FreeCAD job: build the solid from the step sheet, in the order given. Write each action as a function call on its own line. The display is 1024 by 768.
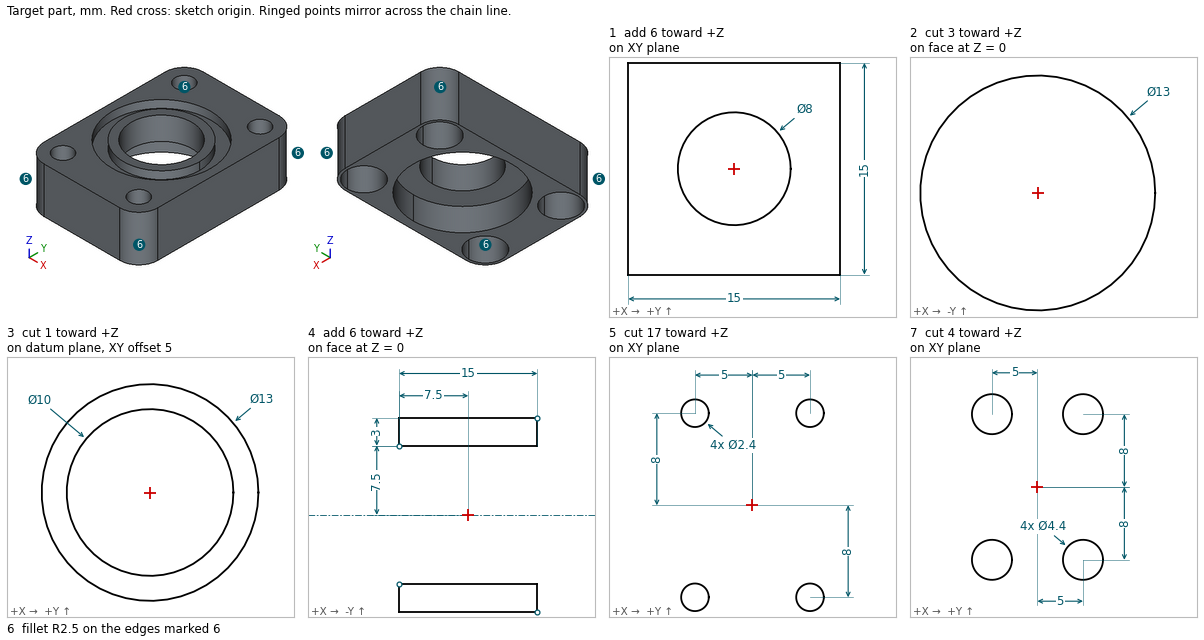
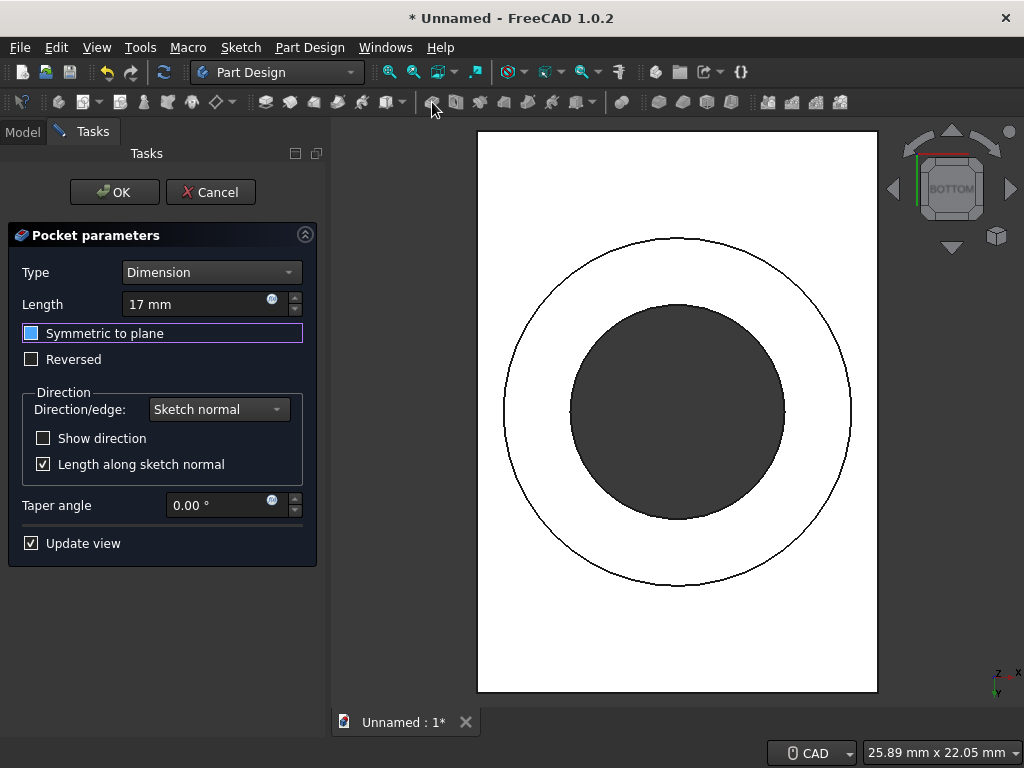
click(30, 359)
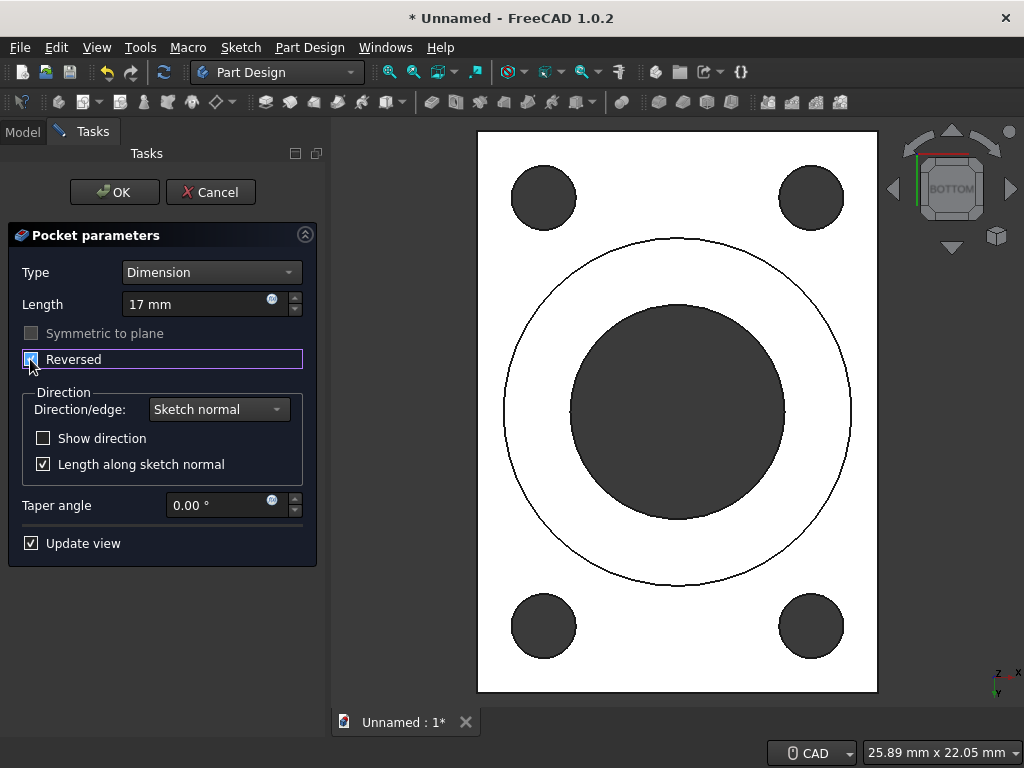
click(115, 192)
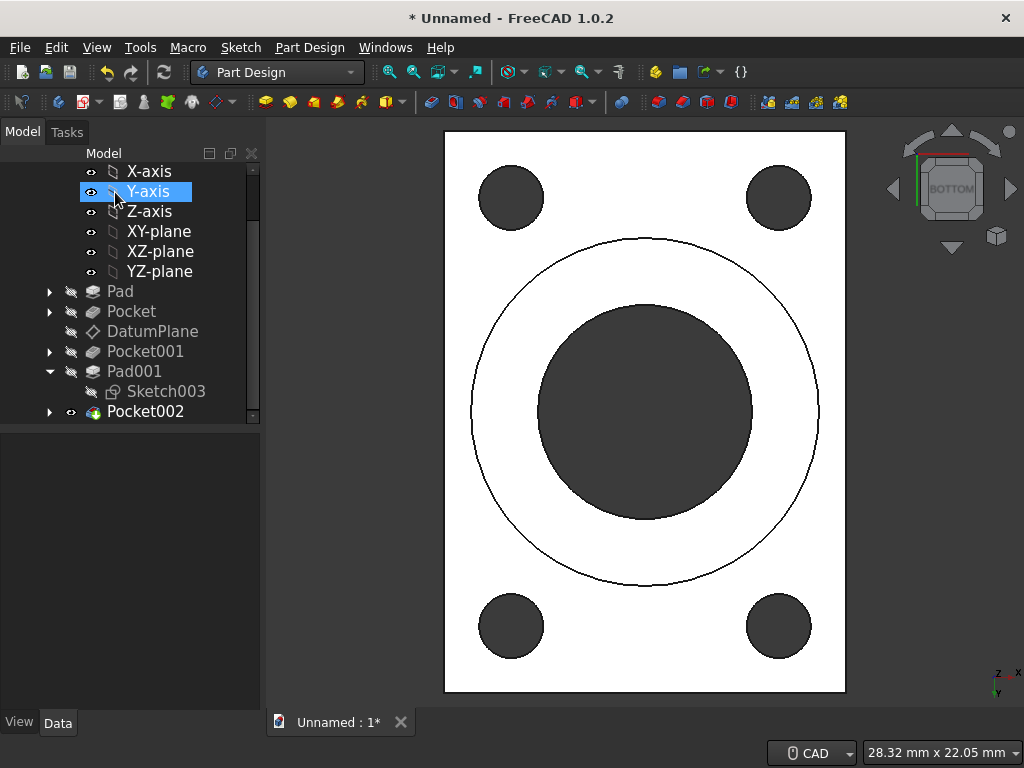
key(0)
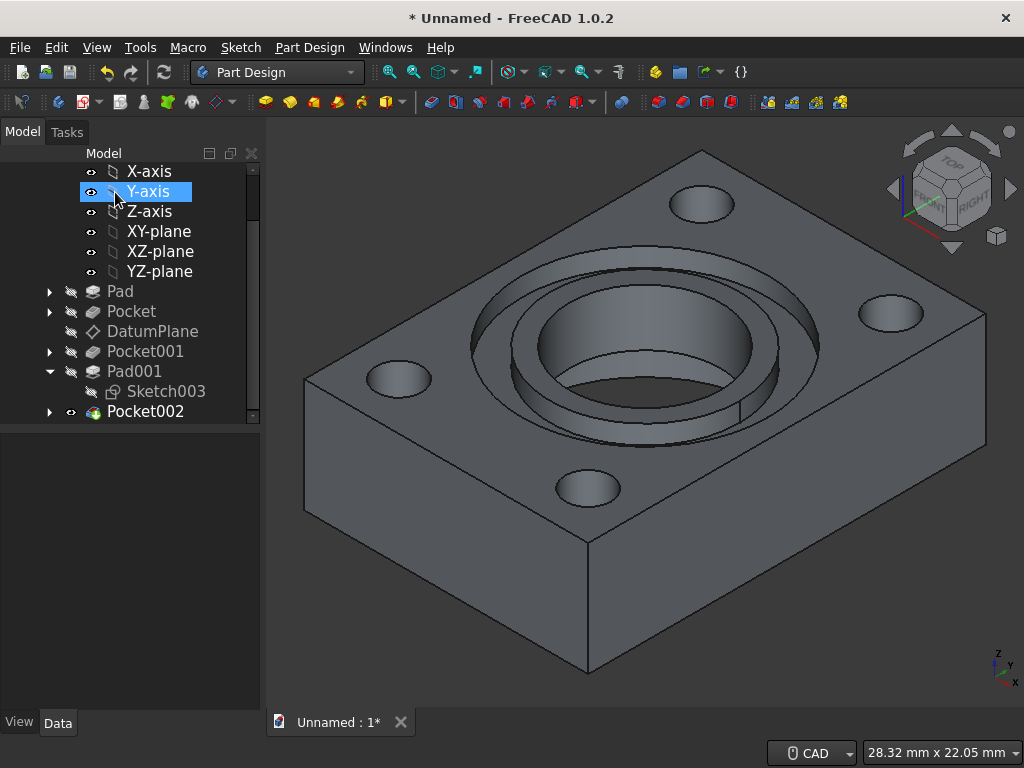
click(588, 608)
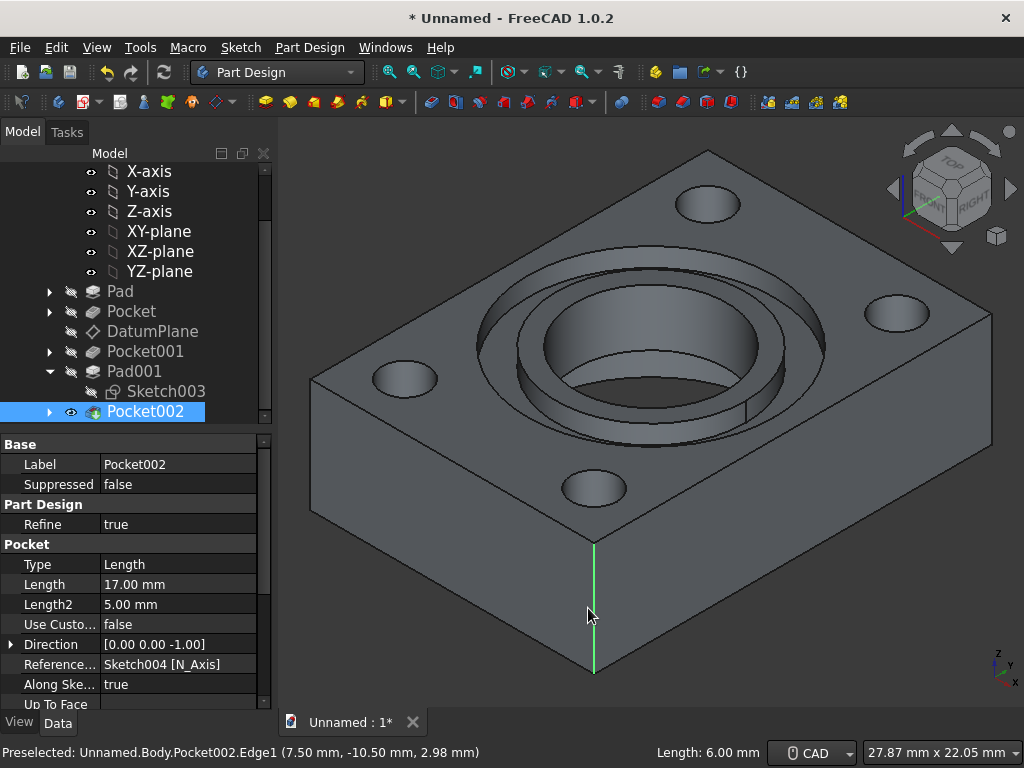
key(2)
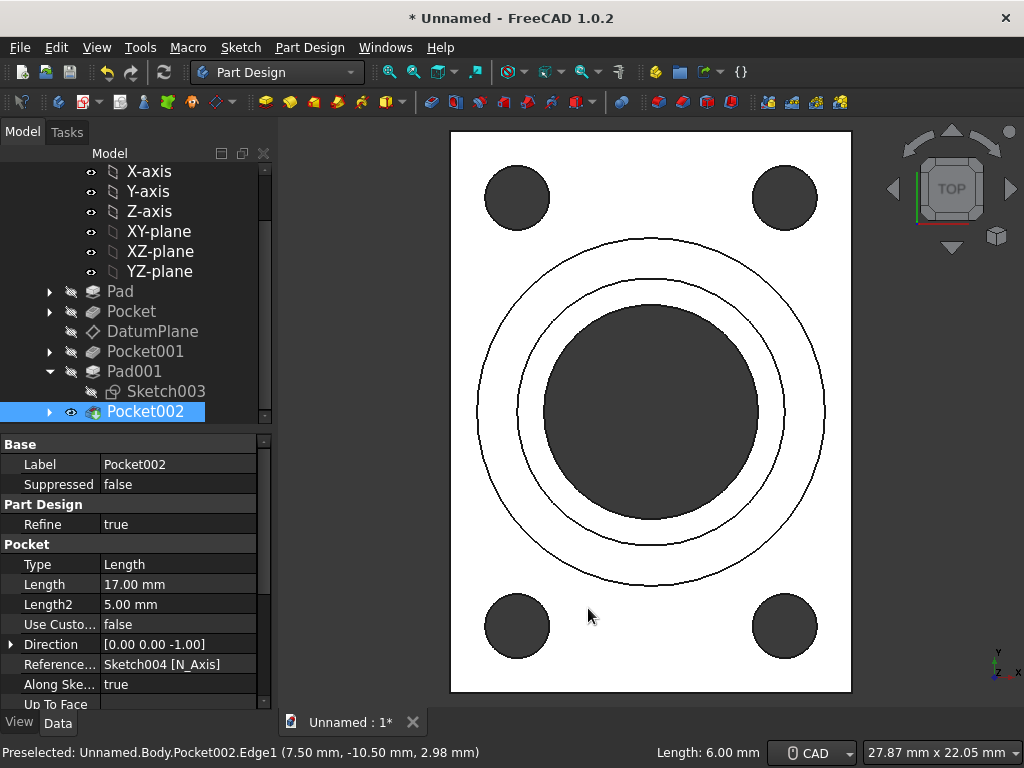
key(1)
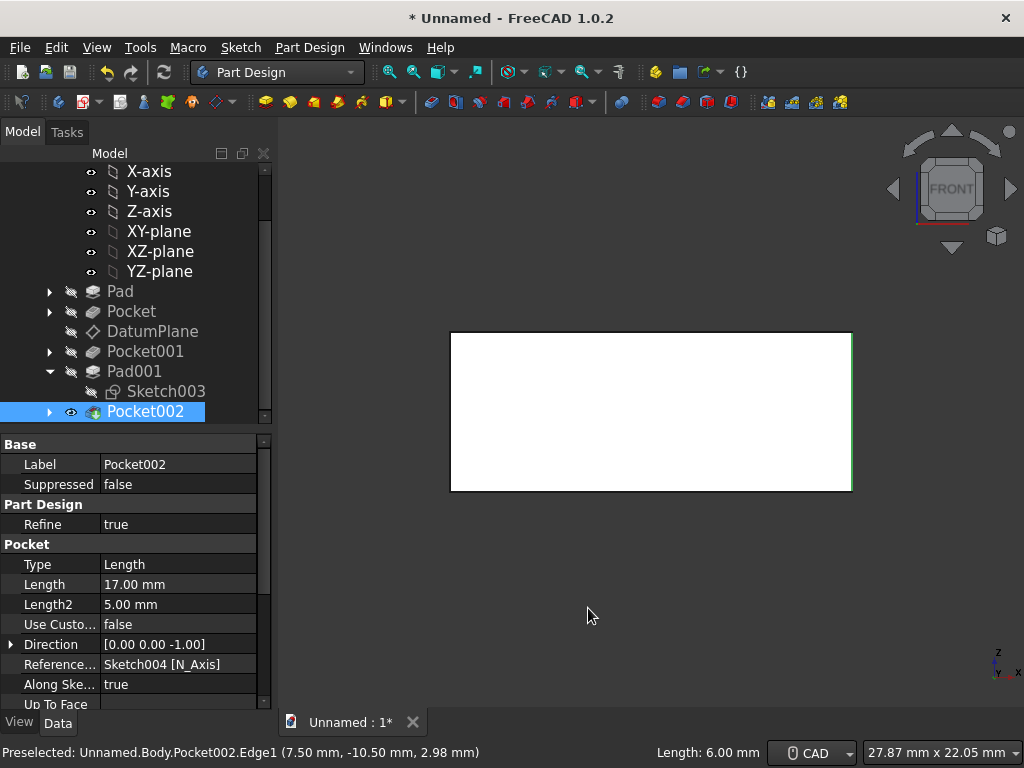
click(450, 411, ctrl)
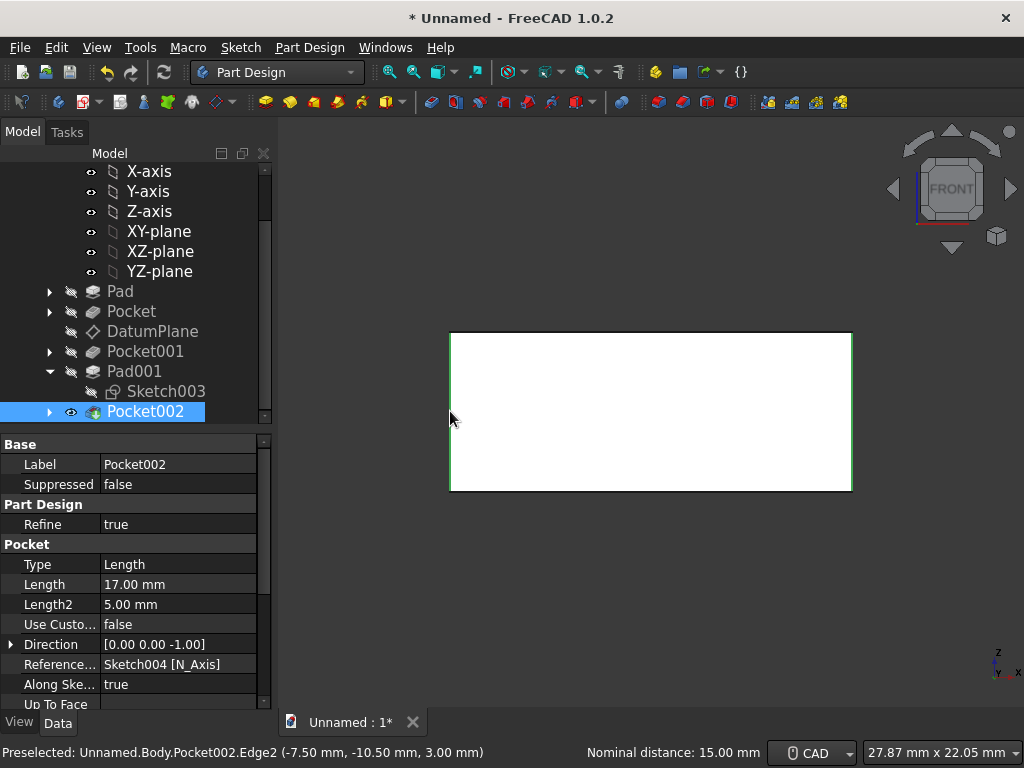
key(3)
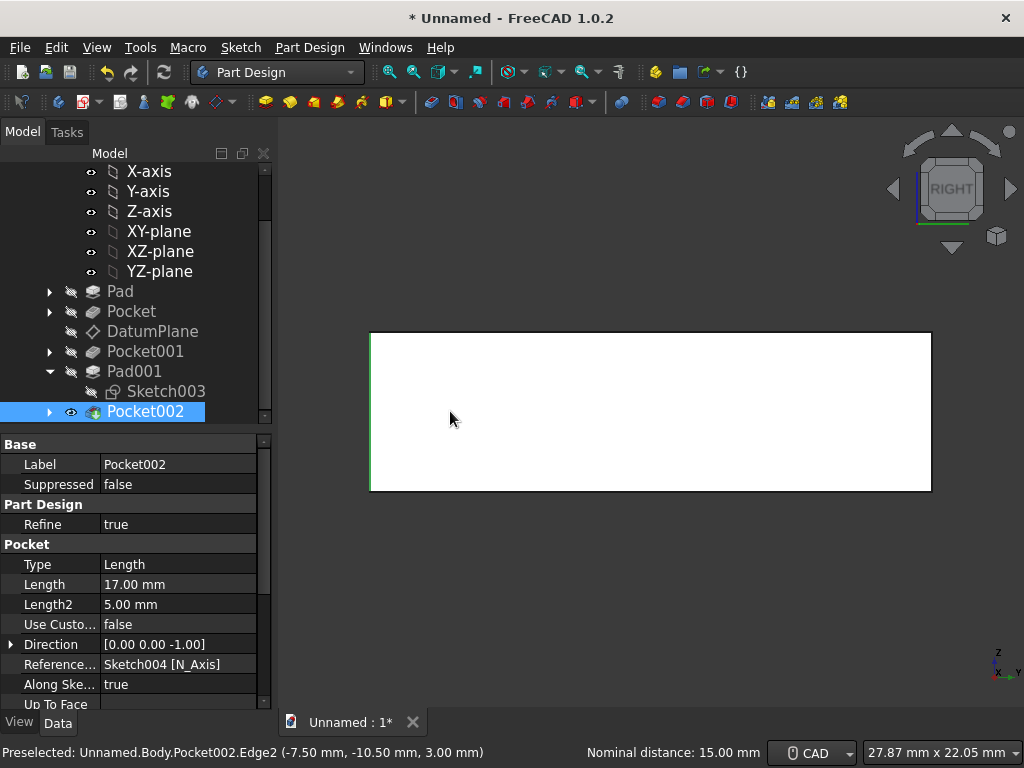
click(932, 411, ctrl)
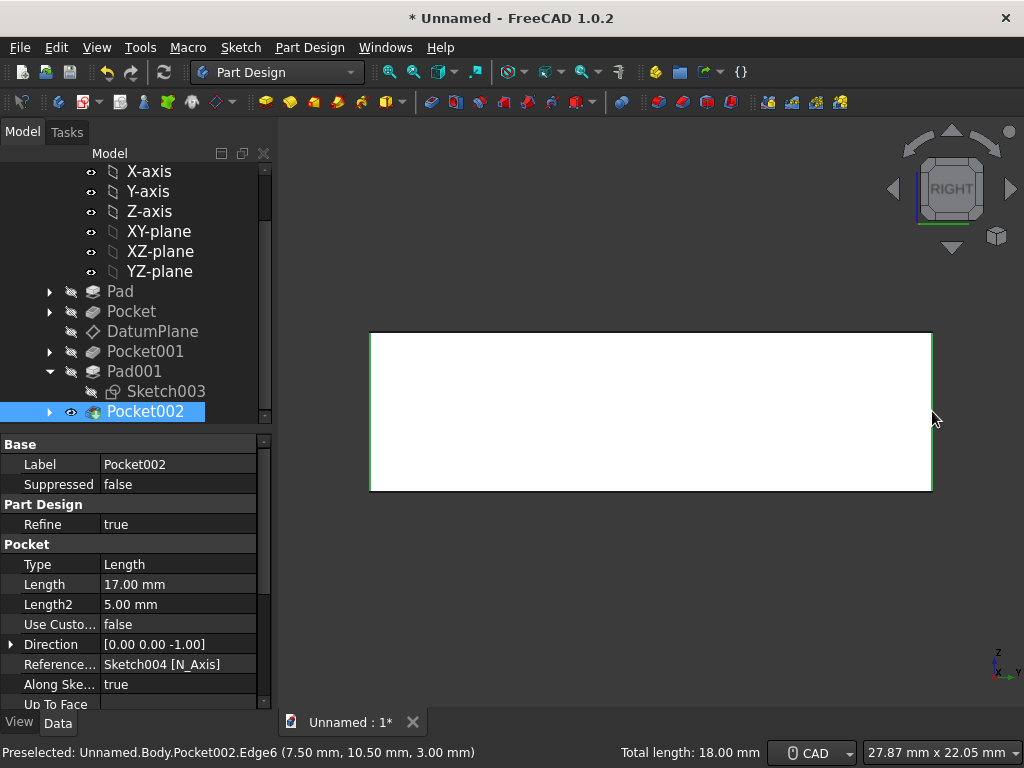
key(5)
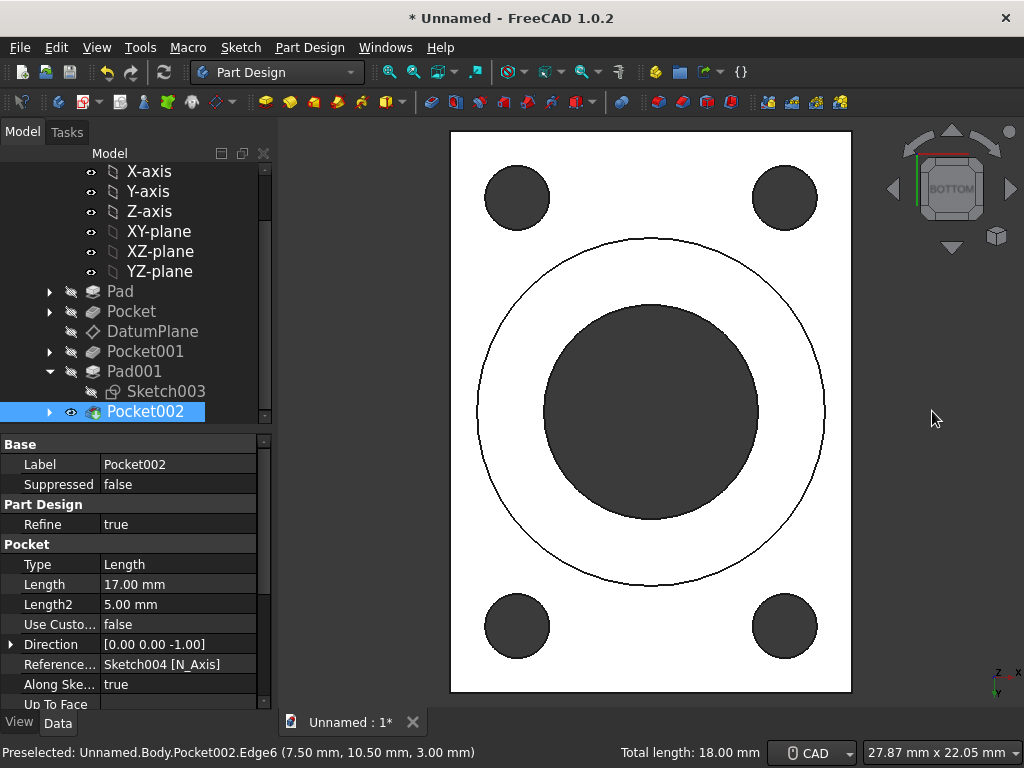
key(4)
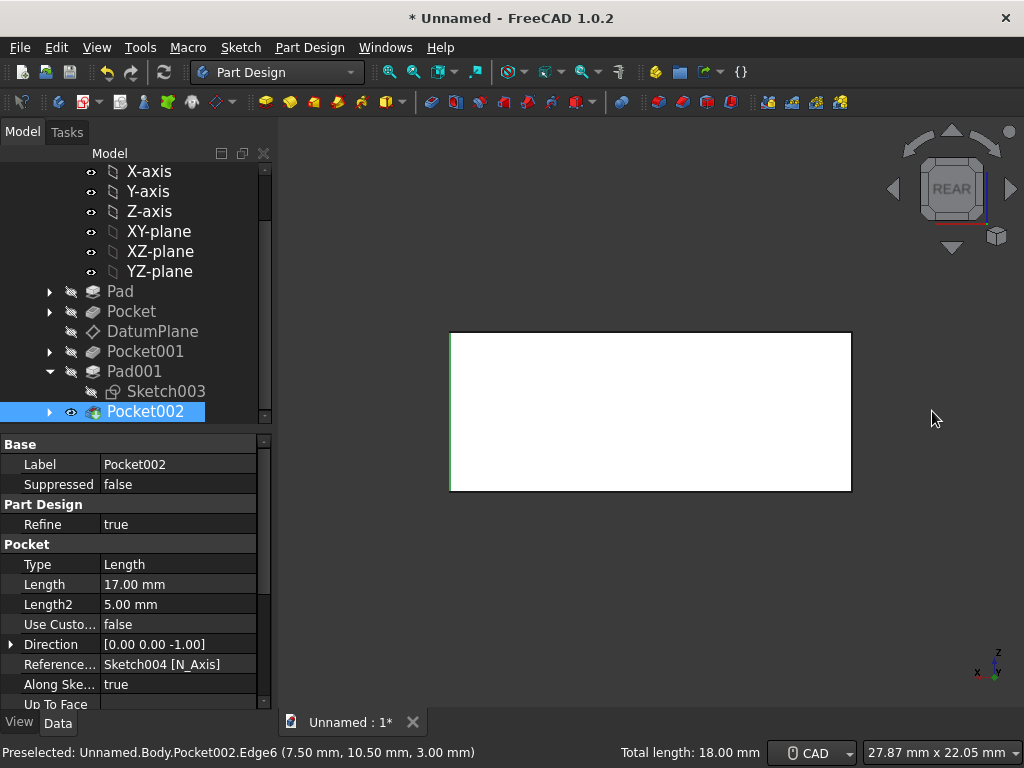
click(852, 411, ctrl)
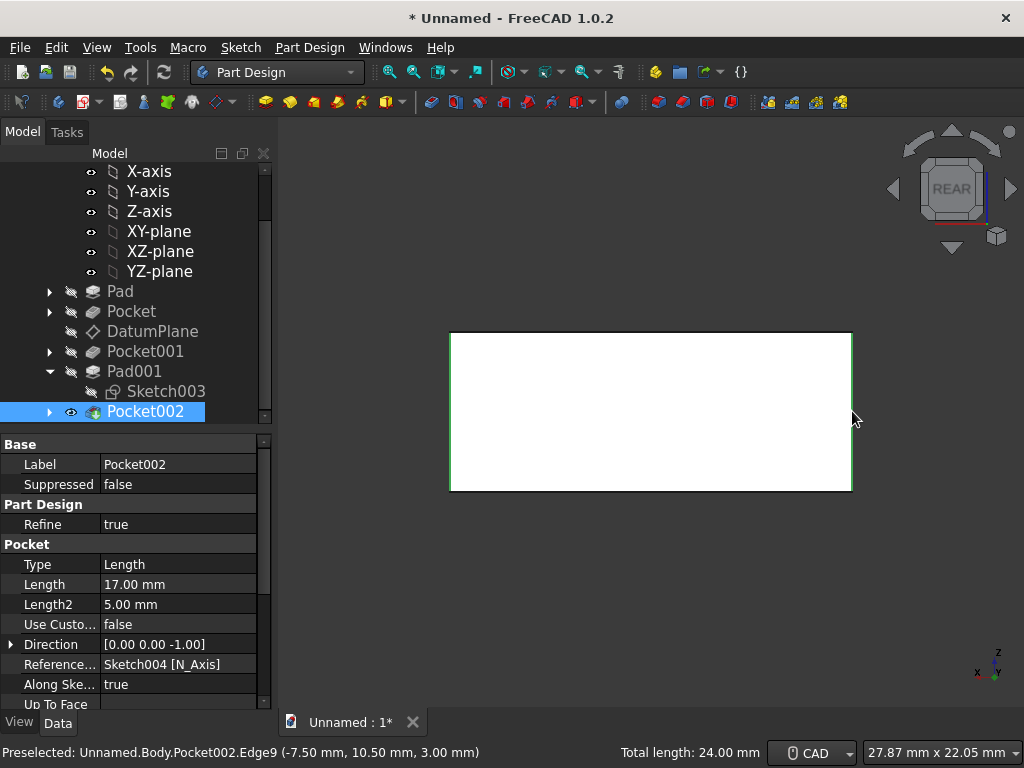
click(660, 102)